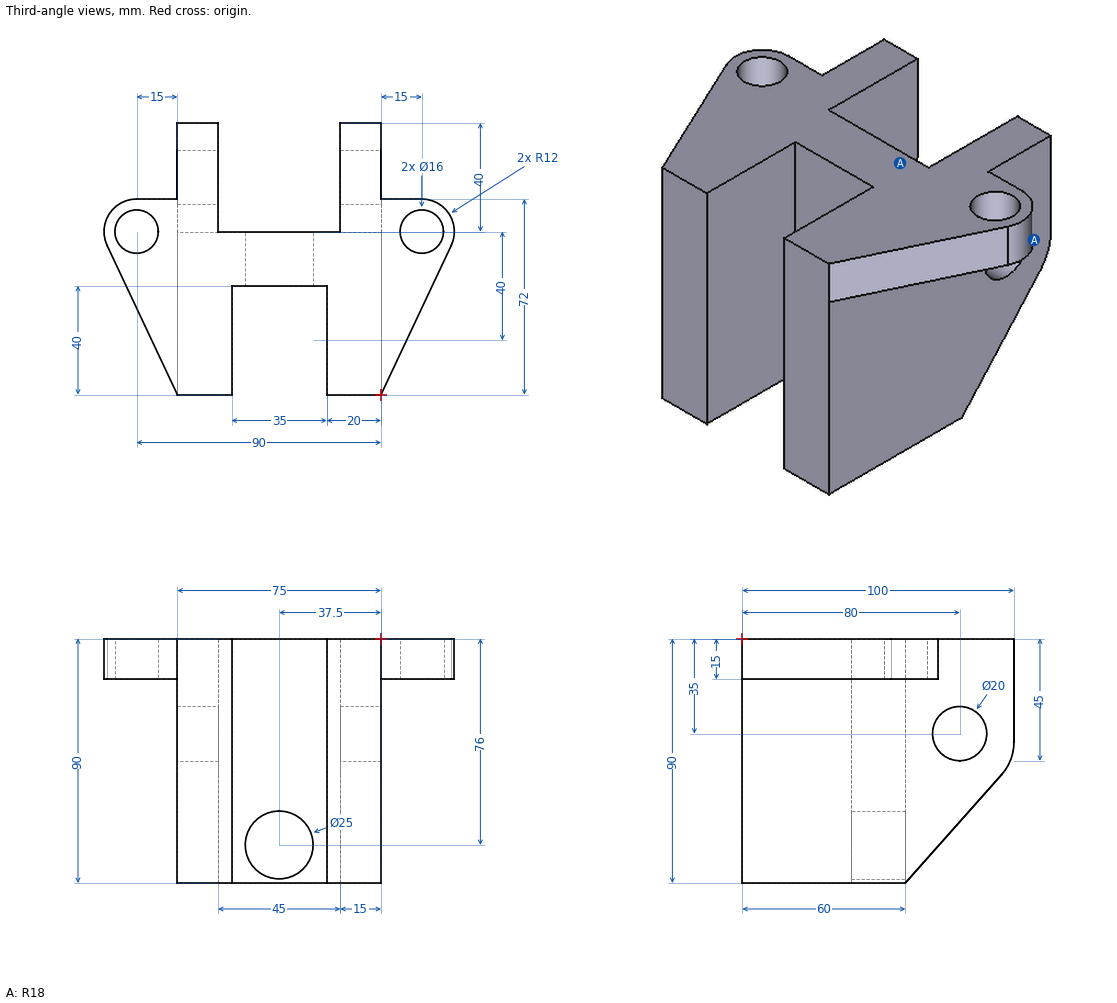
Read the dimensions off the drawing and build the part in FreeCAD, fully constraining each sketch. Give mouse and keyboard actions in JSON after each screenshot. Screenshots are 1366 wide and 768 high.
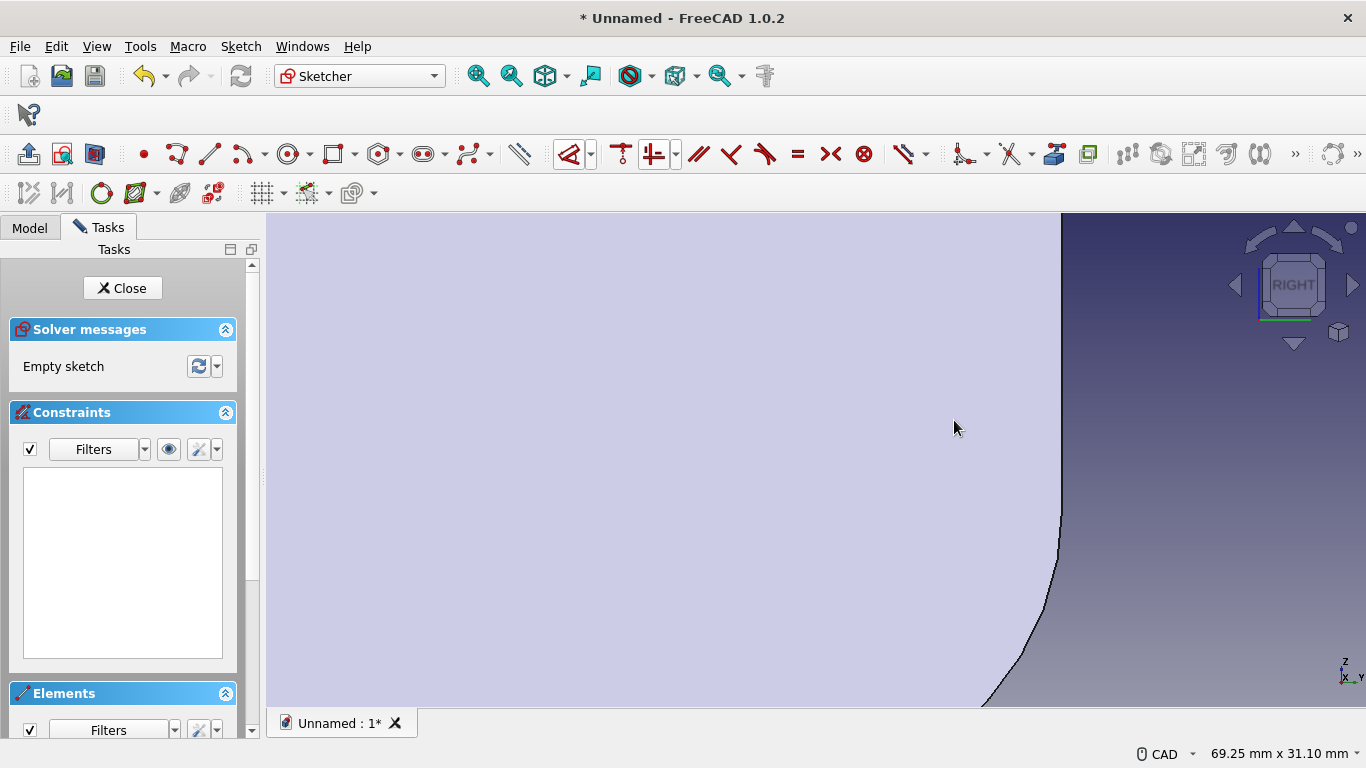
{"action": "left_click", "coordinate": [288, 154]}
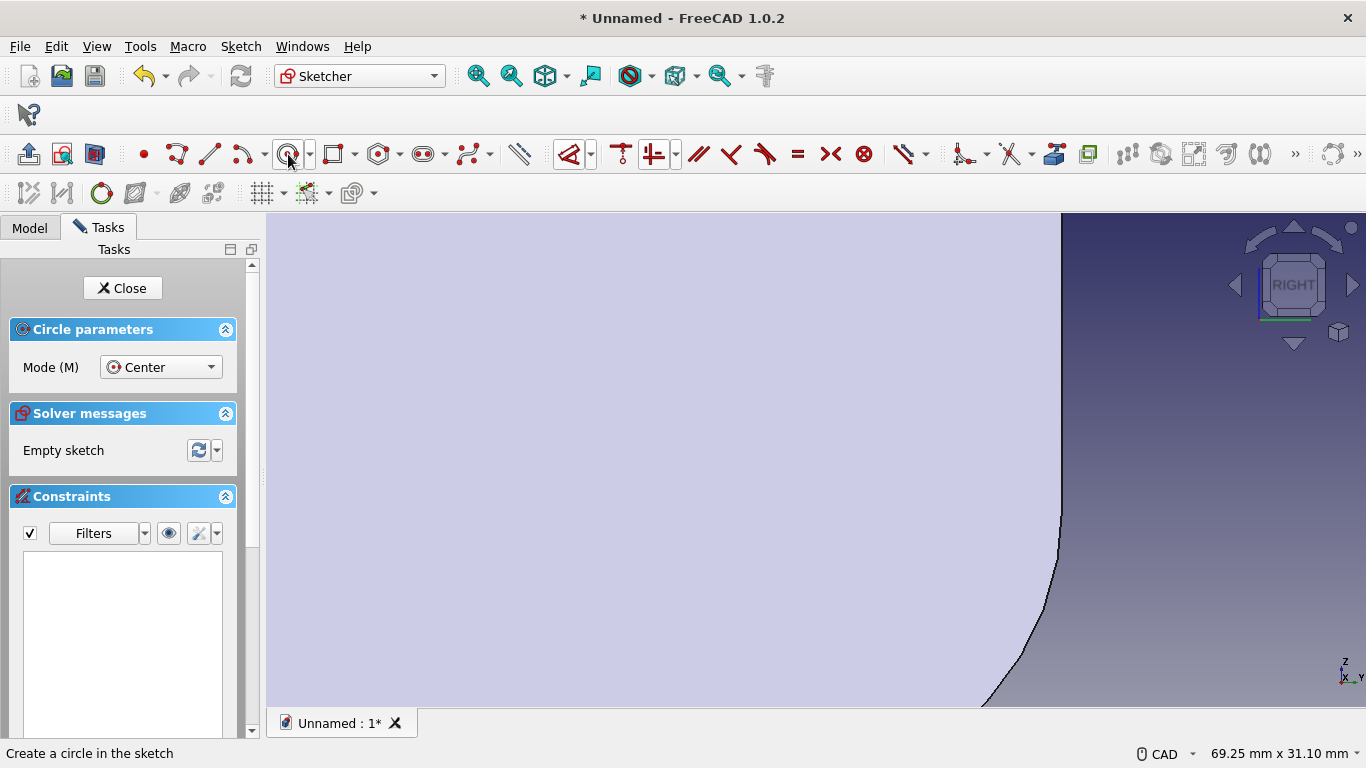
{"action": "left_click", "coordinate": [745, 458]}
{"action": "left_click", "coordinate": [857, 345]}
{"action": "key", "text": "Escape"}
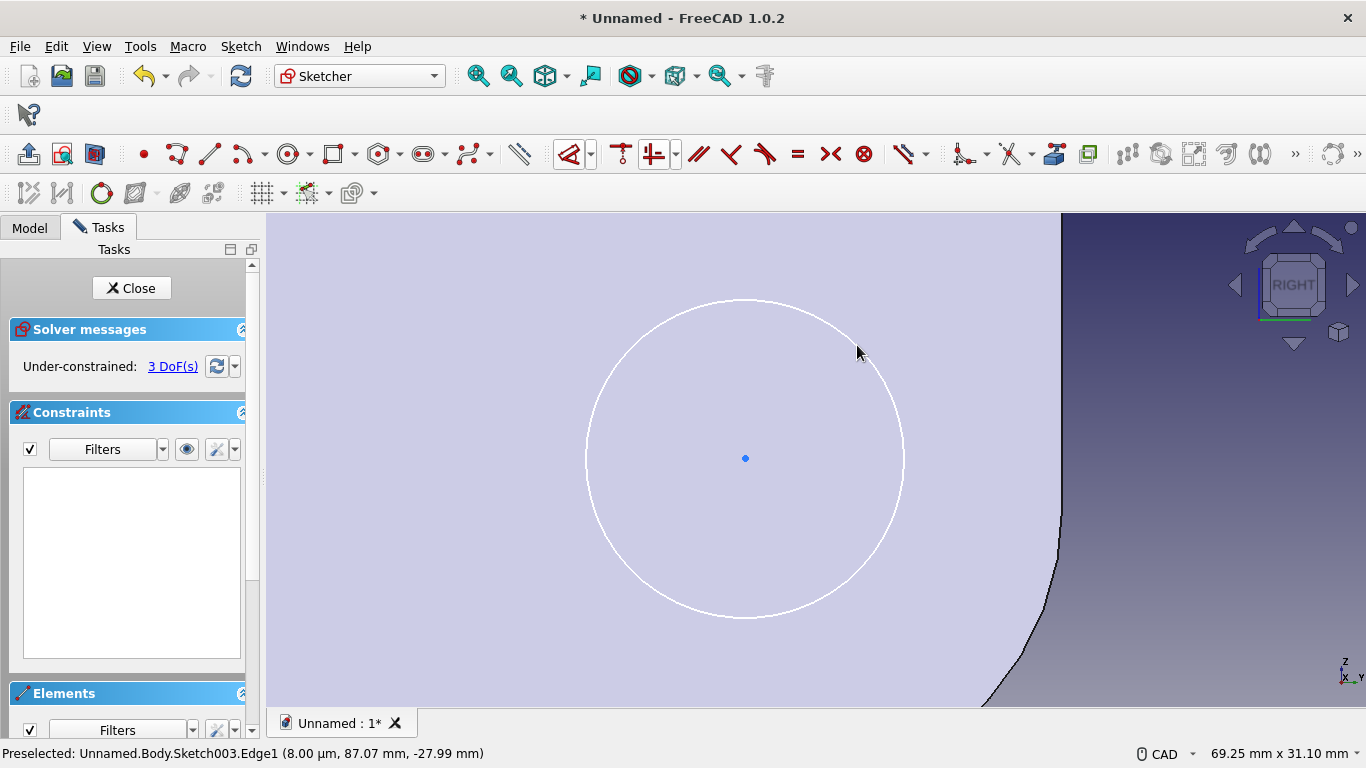
{"action": "left_click", "coordinate": [857, 346]}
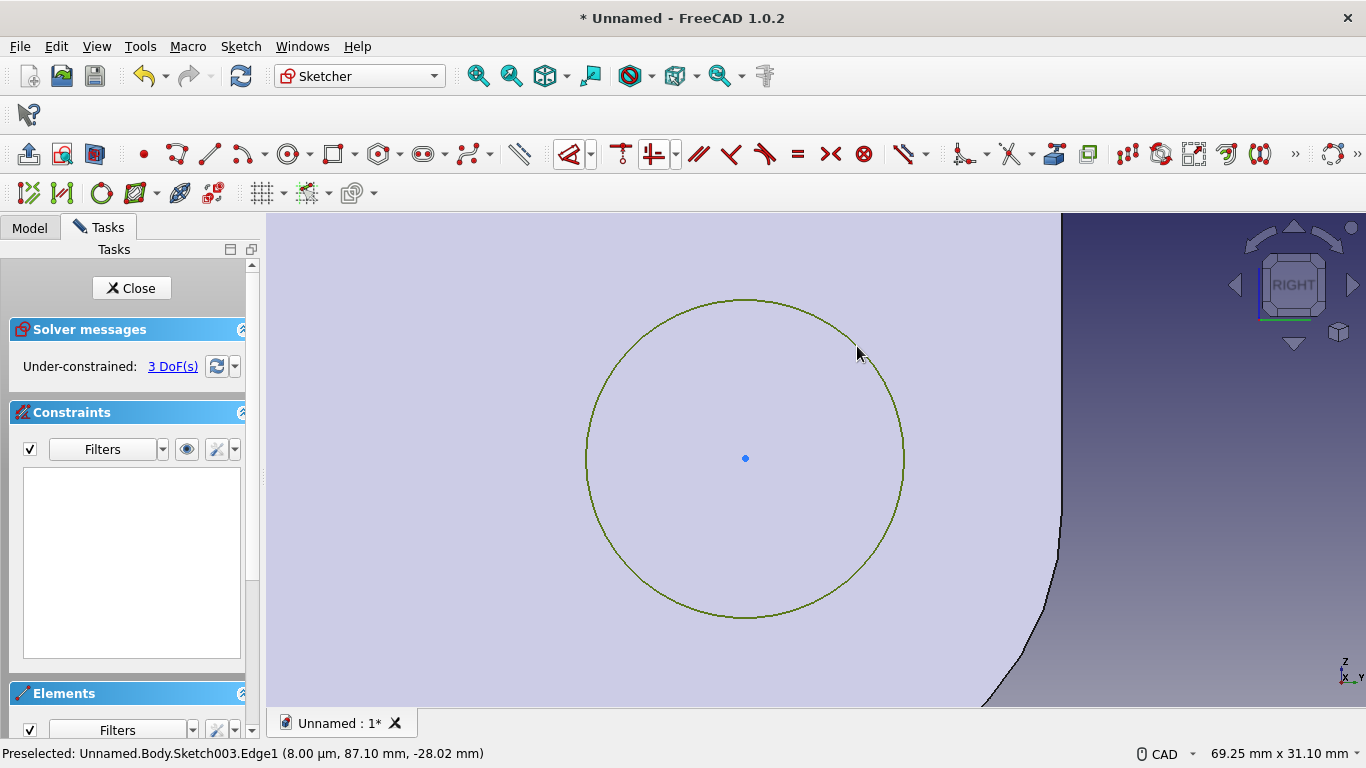
{"action": "left_click", "coordinate": [590, 154]}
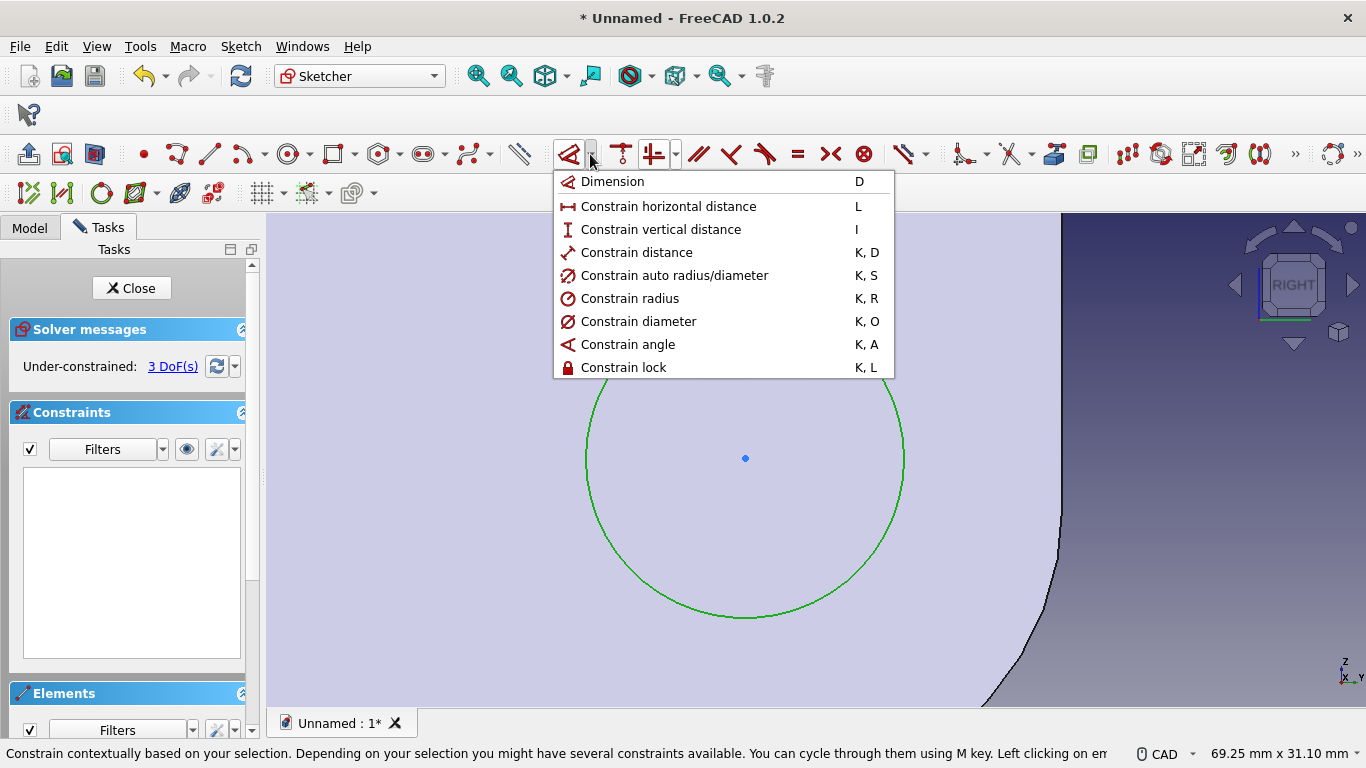
{"action": "left_click", "coordinate": [724, 322]}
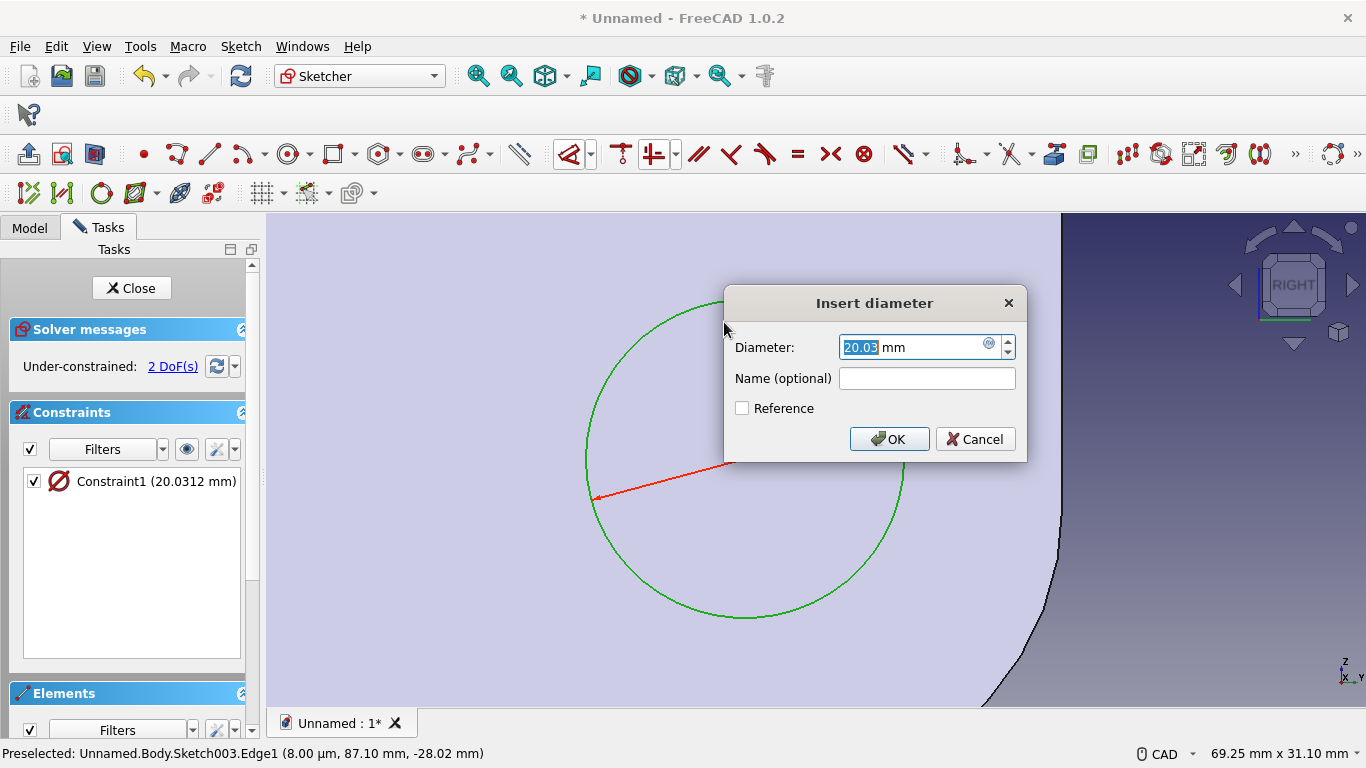
{"action": "type", "text": "20"}
{"action": "key", "text": "Return"}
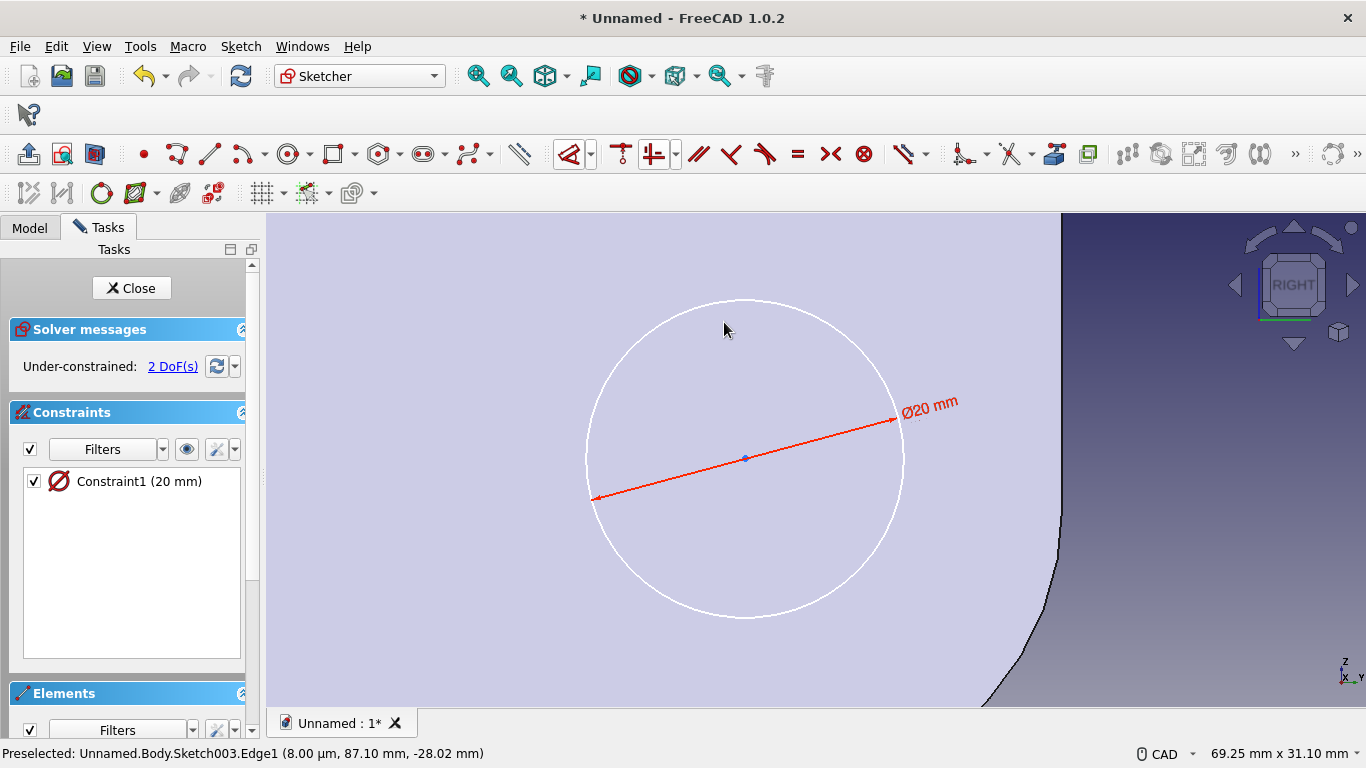
{"action": "left_click", "coordinate": [745, 459]}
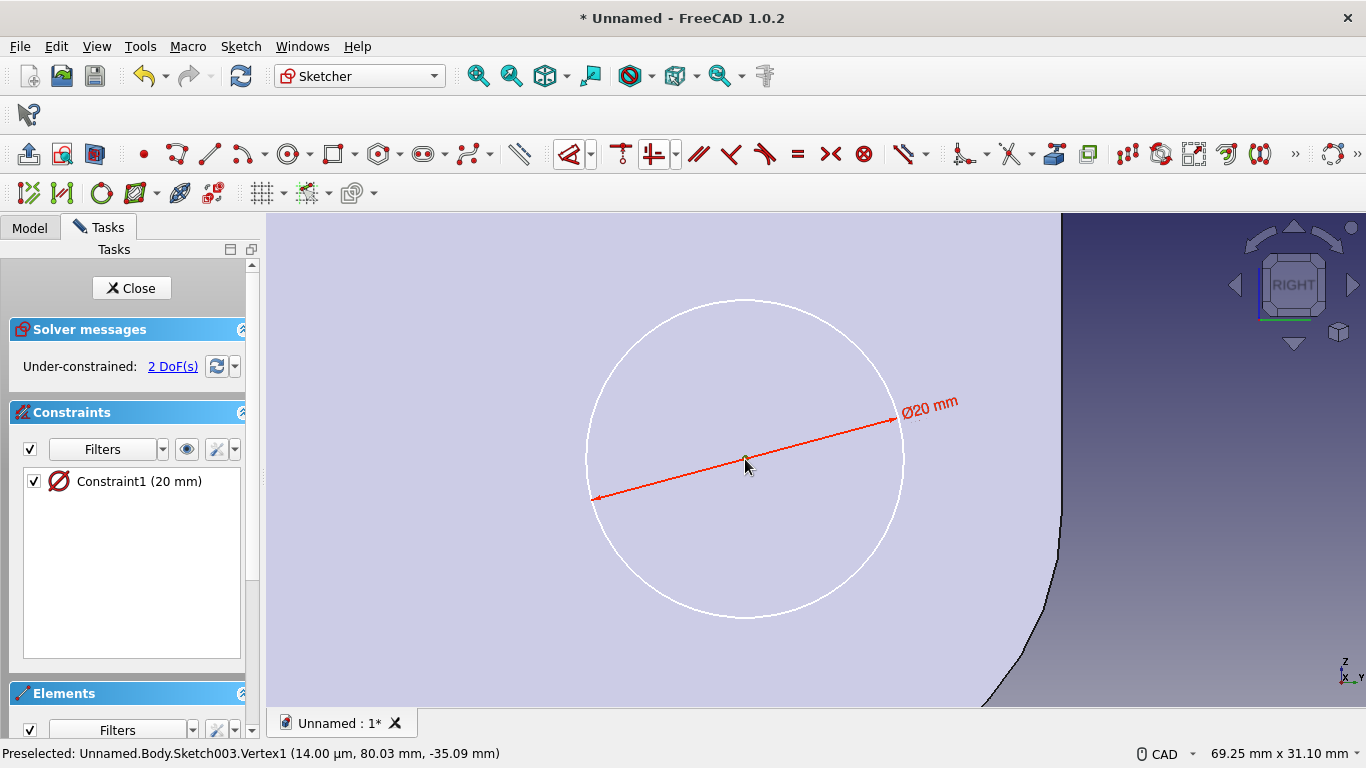
{"action": "left_click", "coordinate": [590, 154]}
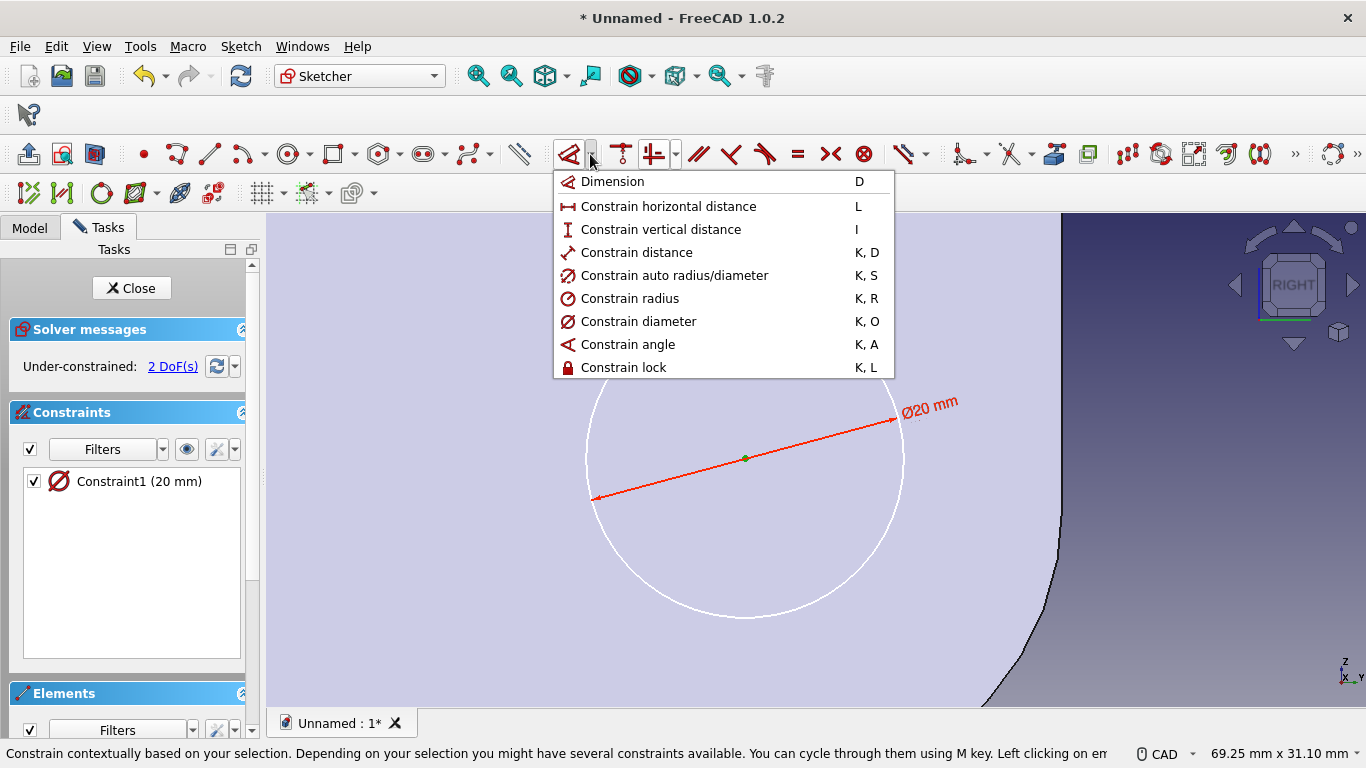
{"action": "left_click", "coordinate": [724, 206]}